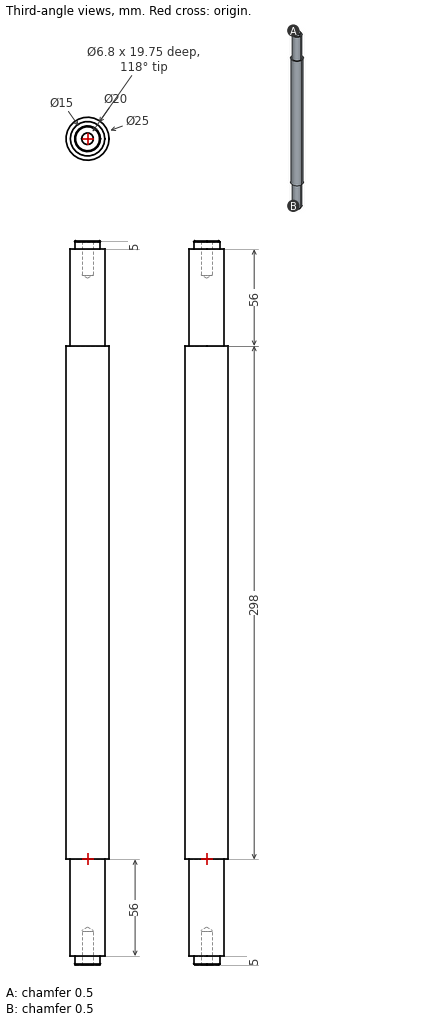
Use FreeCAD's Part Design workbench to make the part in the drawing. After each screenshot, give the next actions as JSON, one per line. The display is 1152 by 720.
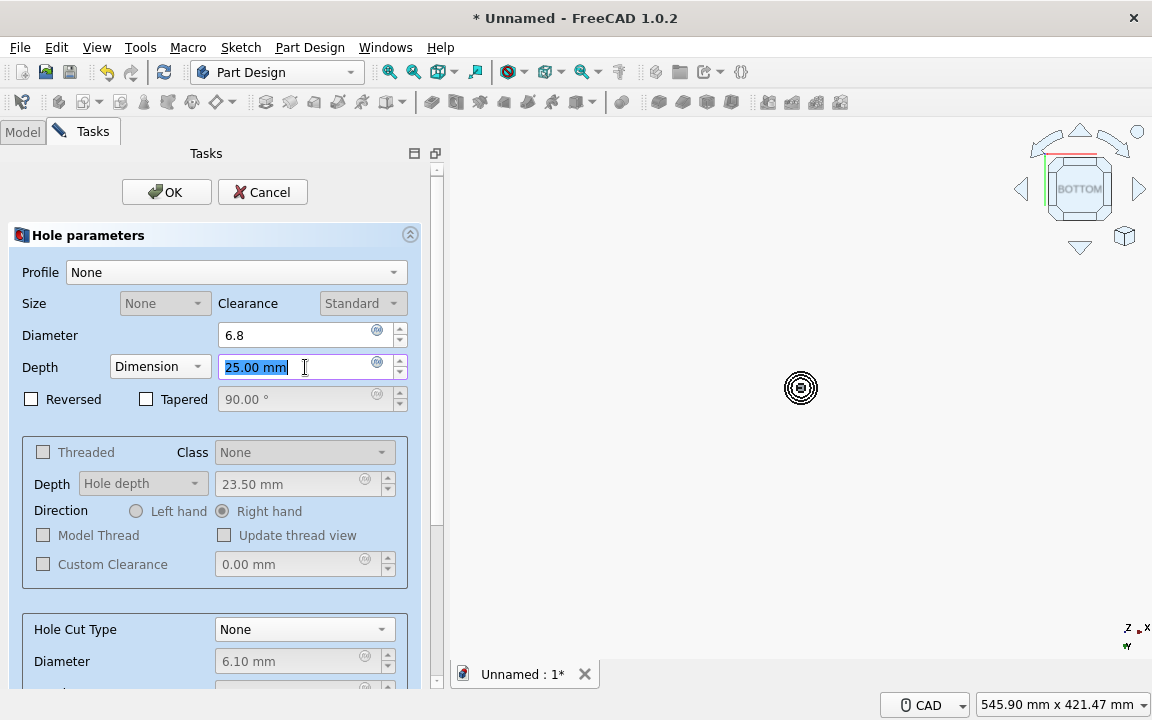
{"action": "type", "text": "19.75"}
{"action": "key", "text": "Tab"}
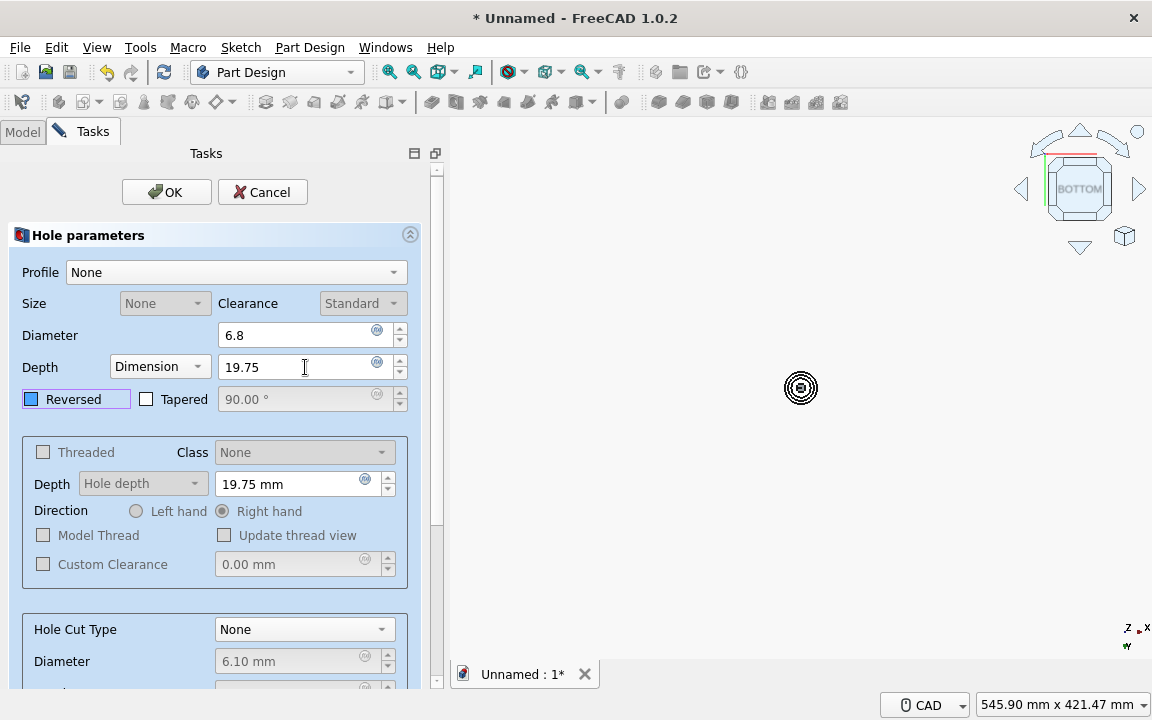
{"action": "left_click", "coordinate": [167, 192]}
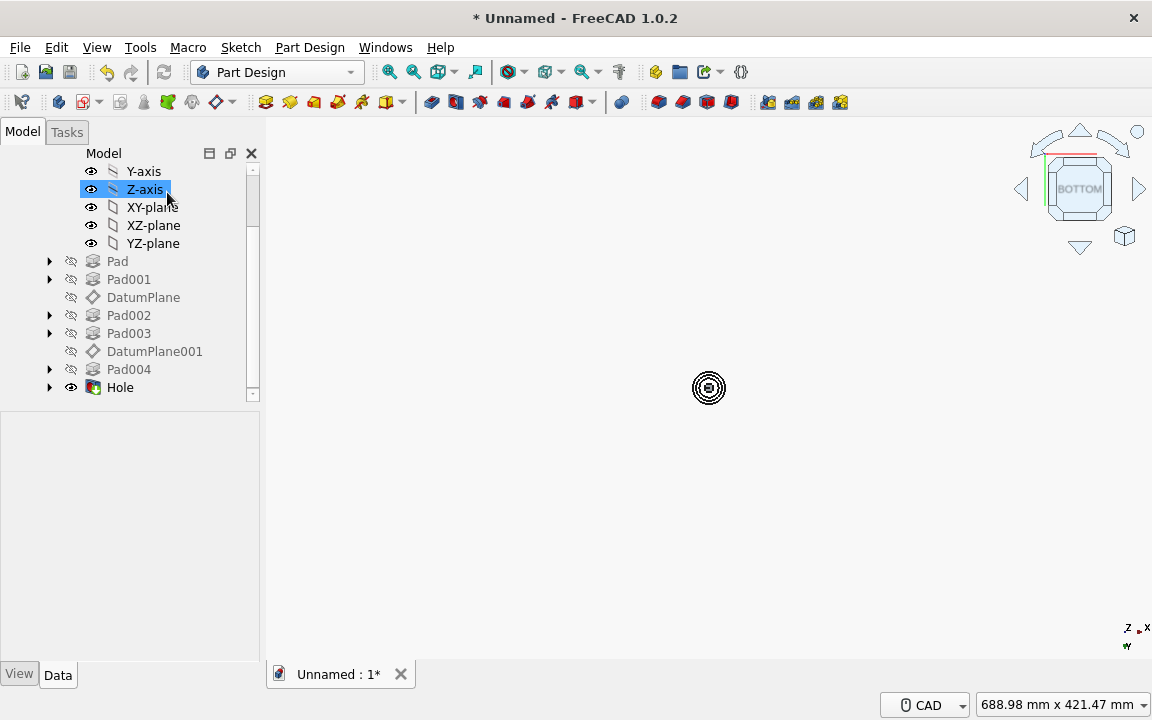
{"action": "left_click", "coordinate": [390, 72]}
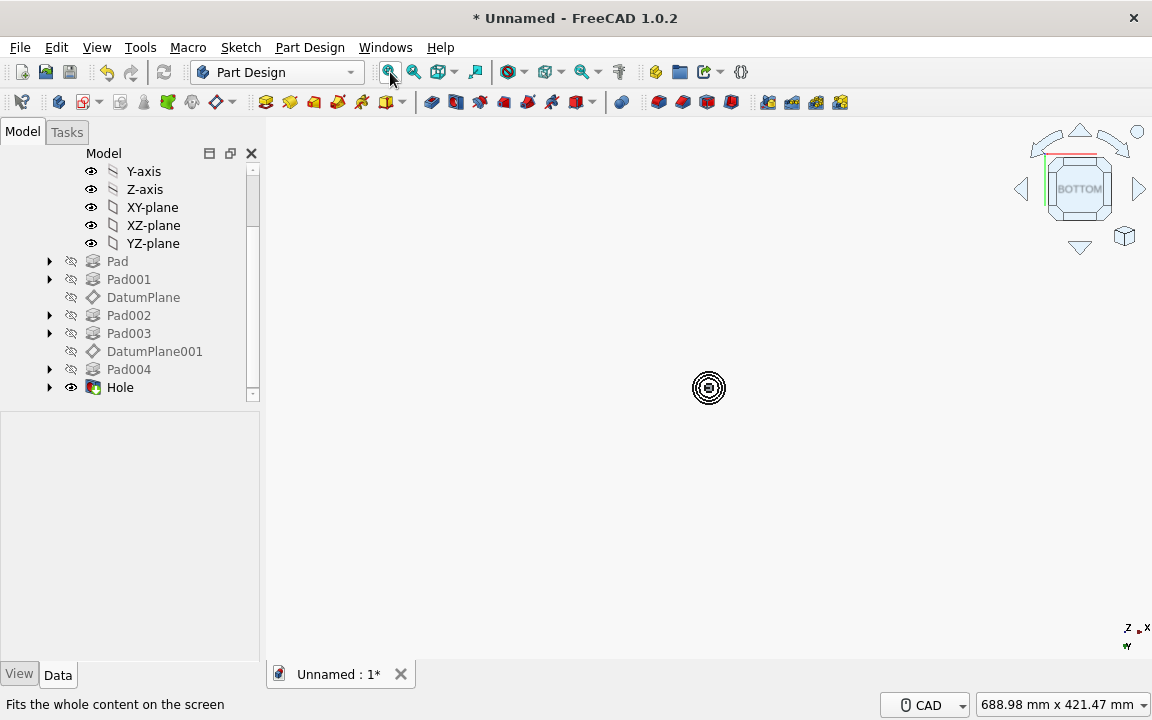
{"action": "key", "text": "0"}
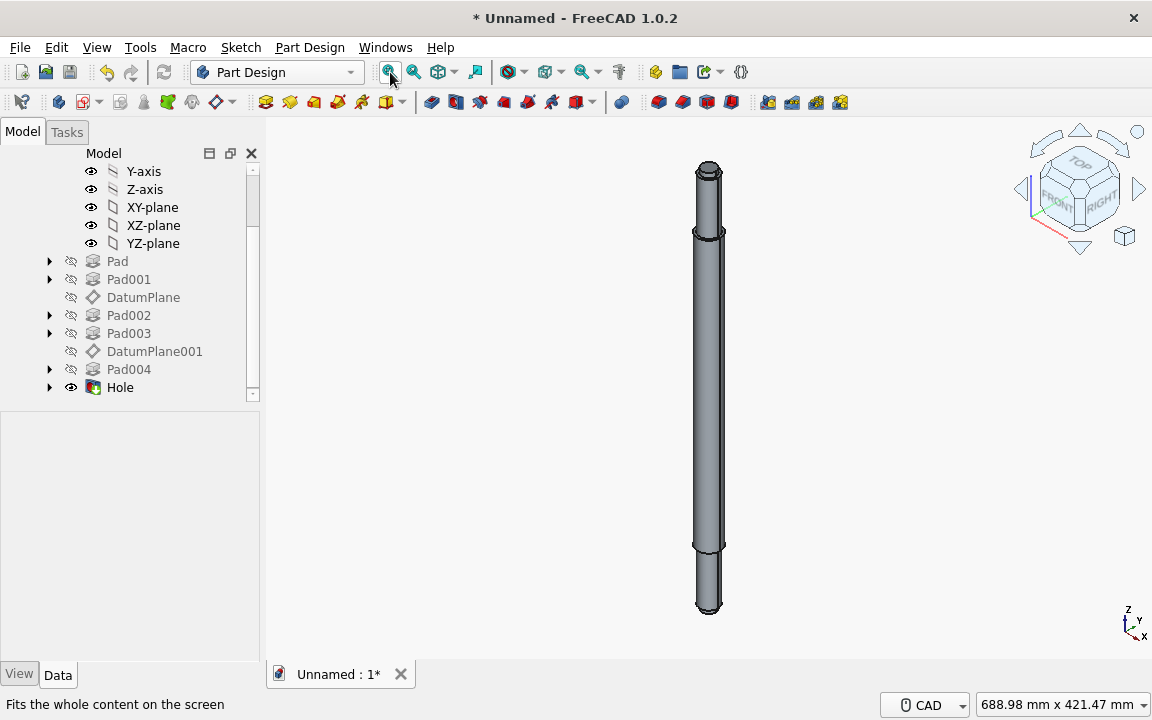
{"action": "key", "text": "2"}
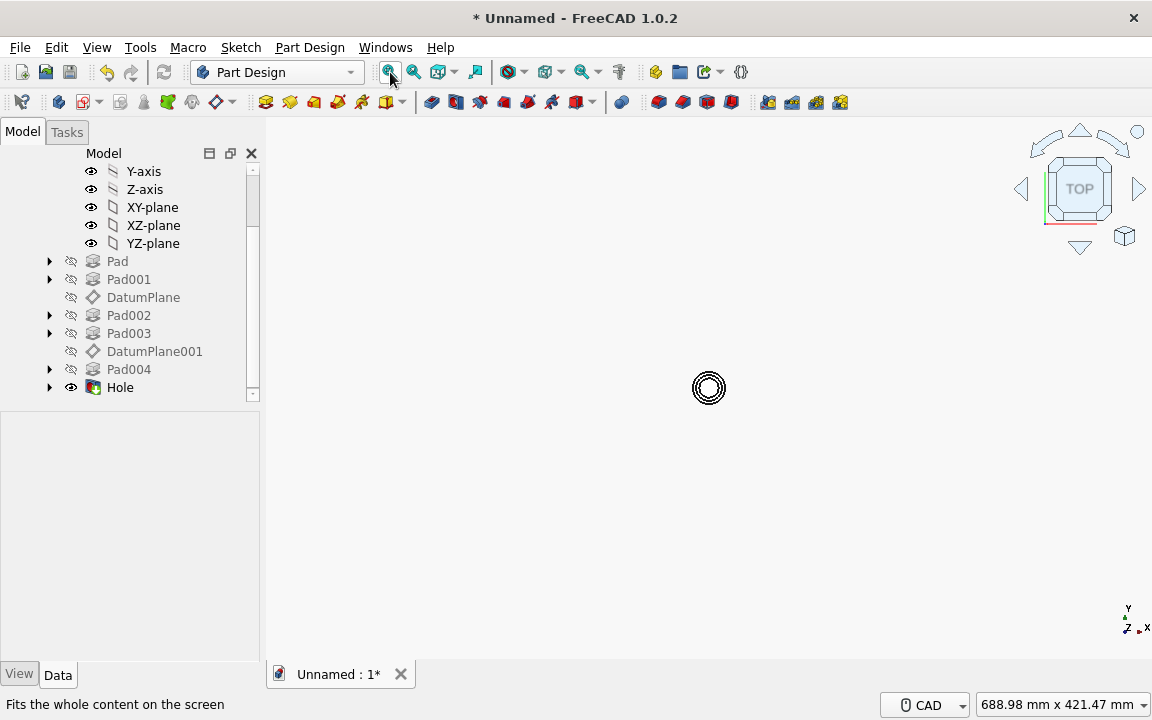
{"action": "left_click", "coordinate": [390, 72]}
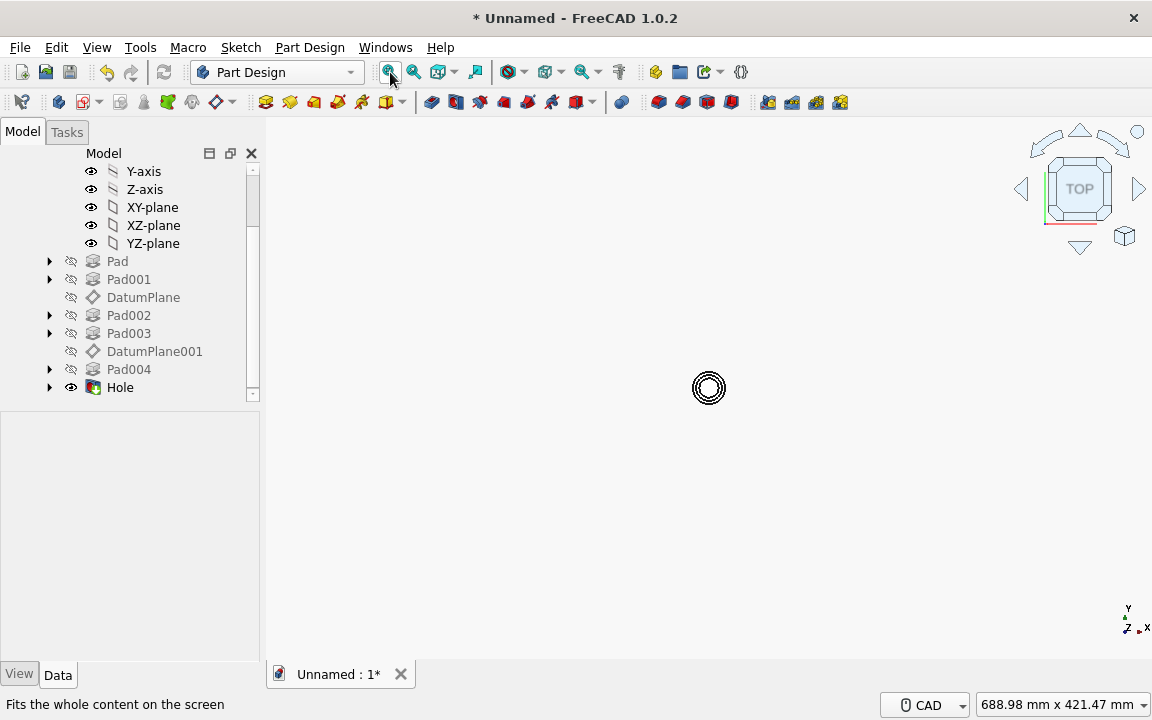
{"action": "left_click", "coordinate": [709, 387]}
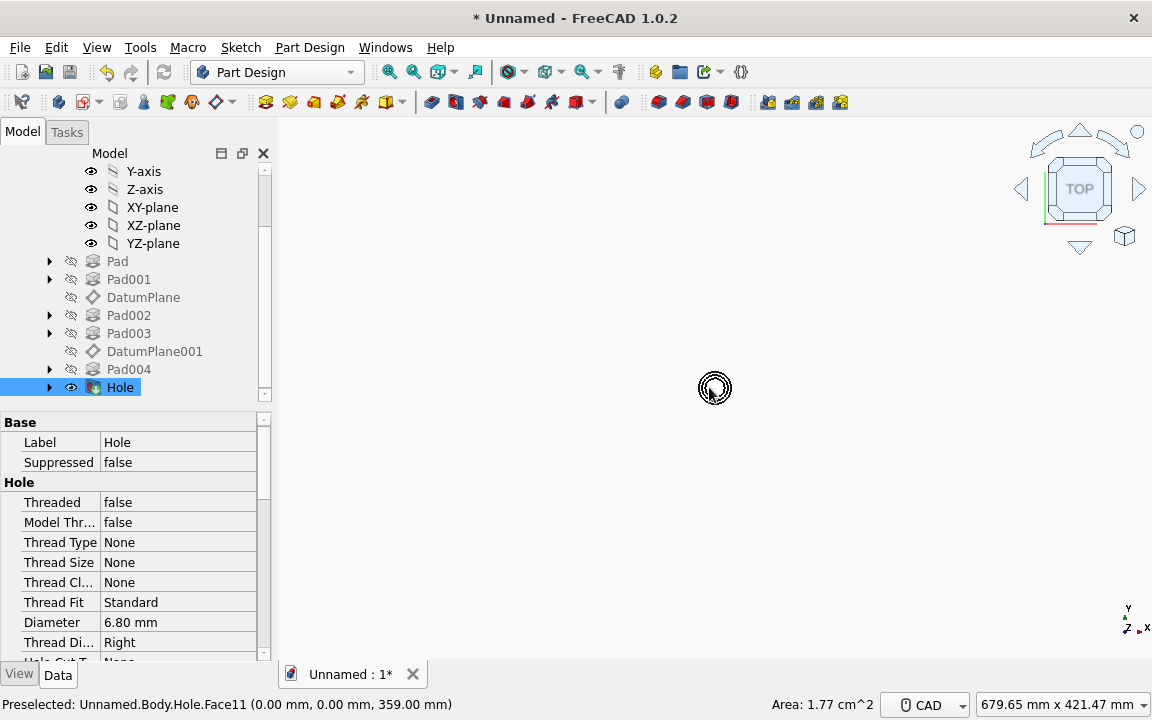
{"action": "left_click", "coordinate": [84, 102]}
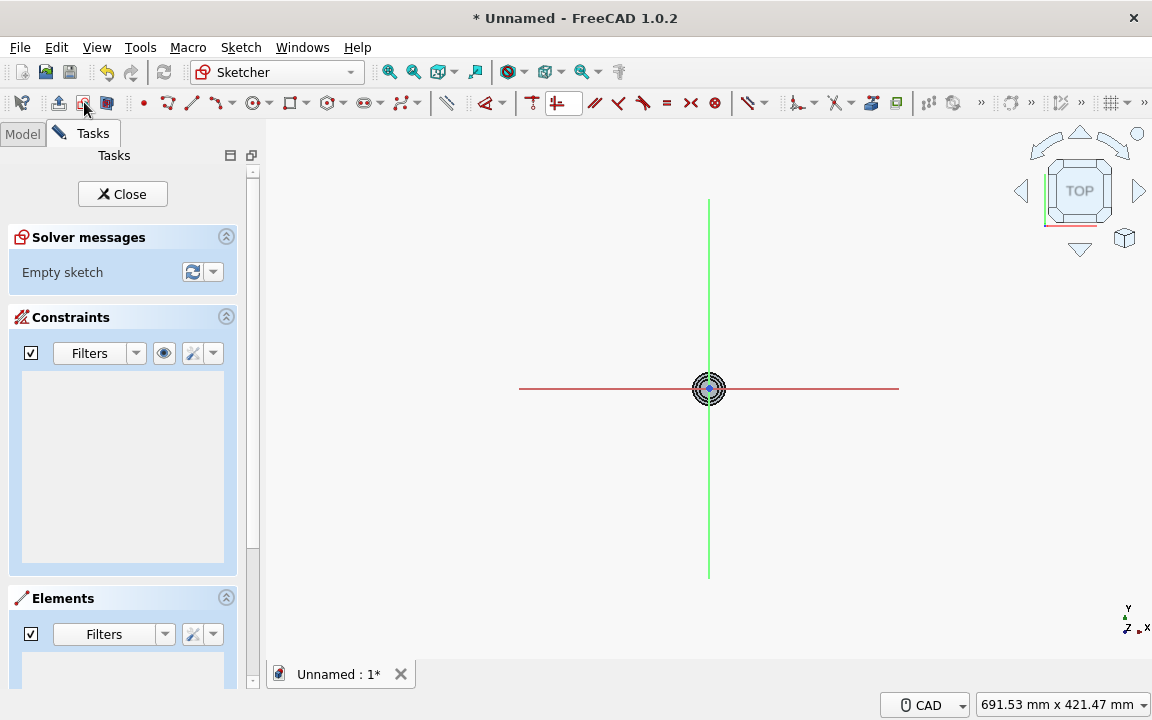
{"action": "scroll", "coordinate": [713, 389], "scroll_direction": "up", "scroll_amount": 15}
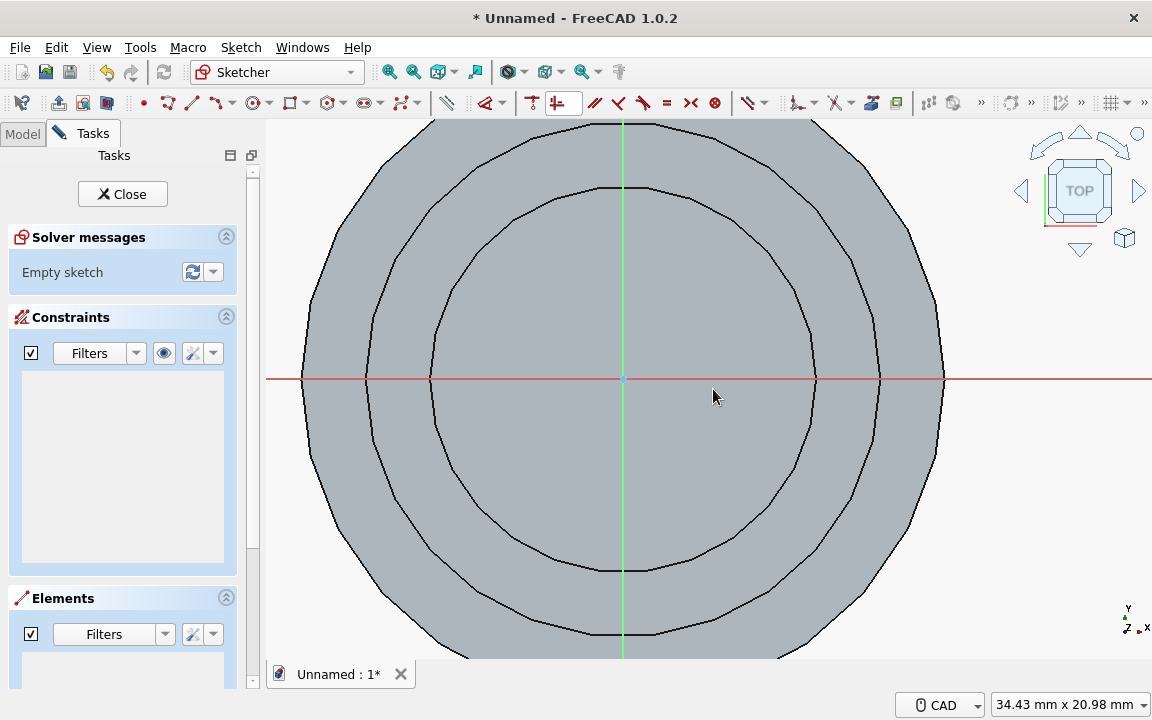
{"action": "scroll", "coordinate": [602, 368], "scroll_direction": "up", "scroll_amount": 3}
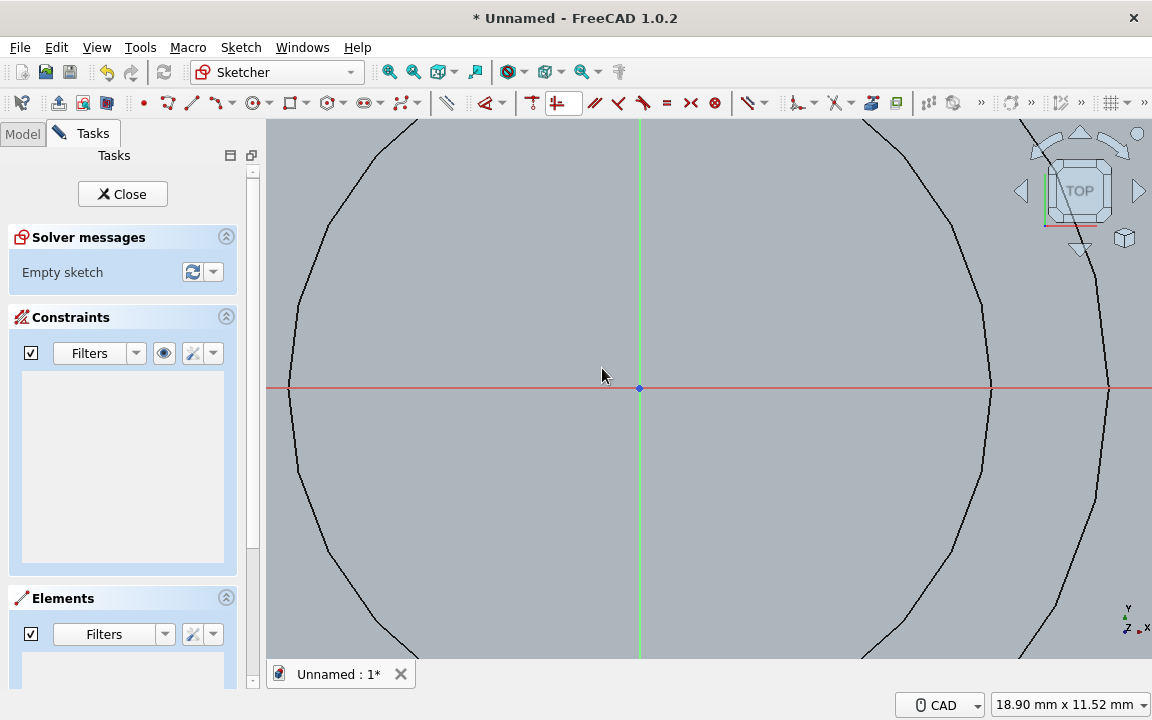
{"action": "left_click", "coordinate": [254, 104]}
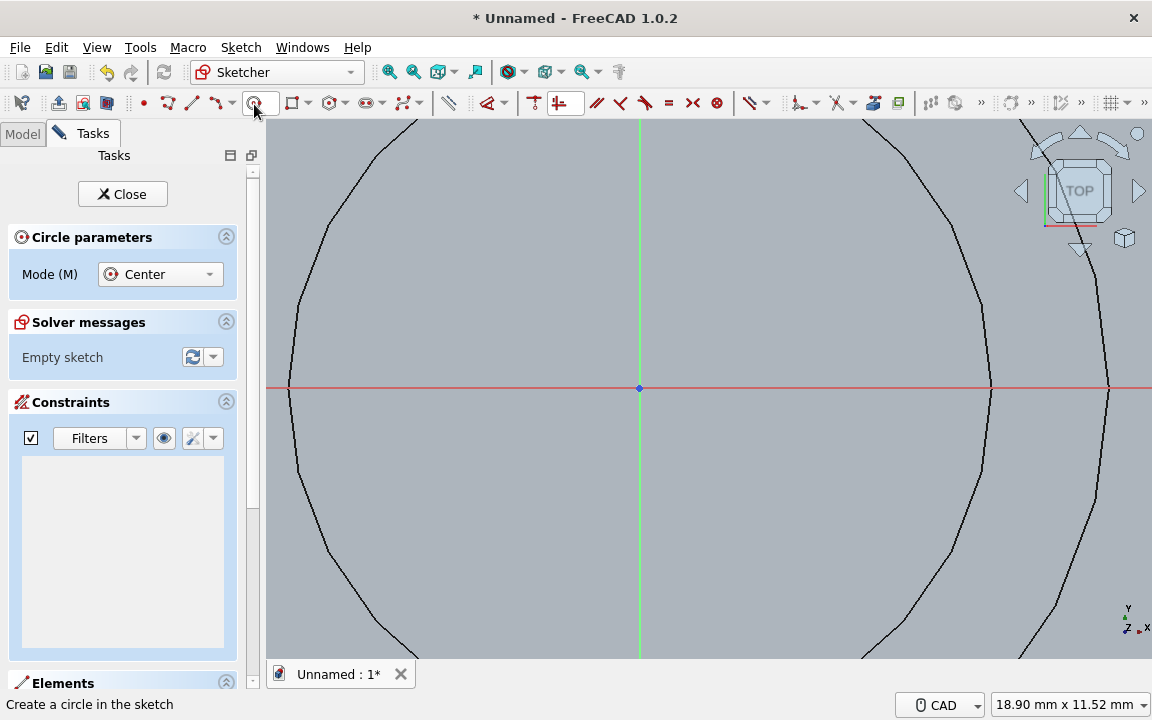
{"action": "left_click", "coordinate": [640, 388]}
{"action": "left_click", "coordinate": [753, 276]}
{"action": "key", "text": "Escape"}